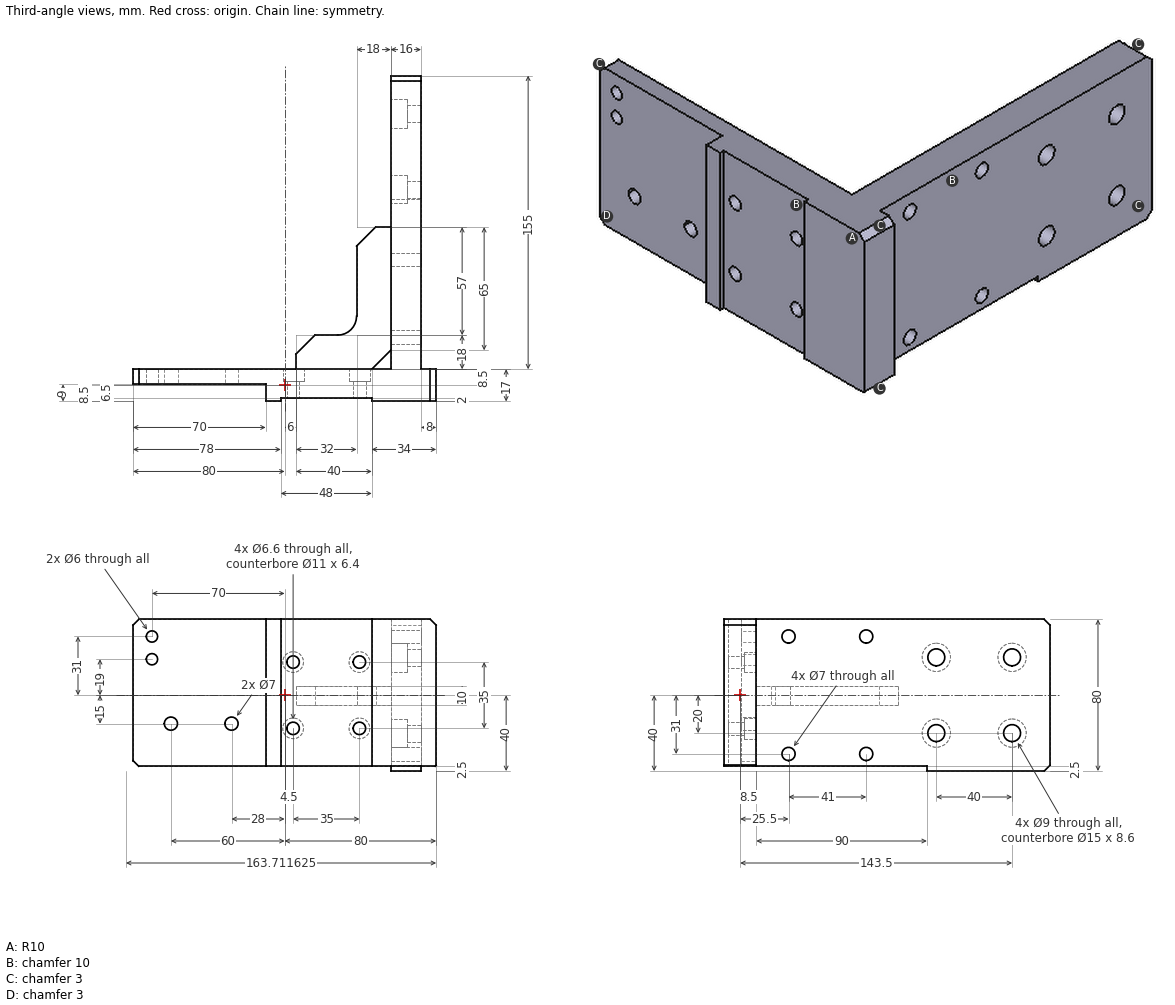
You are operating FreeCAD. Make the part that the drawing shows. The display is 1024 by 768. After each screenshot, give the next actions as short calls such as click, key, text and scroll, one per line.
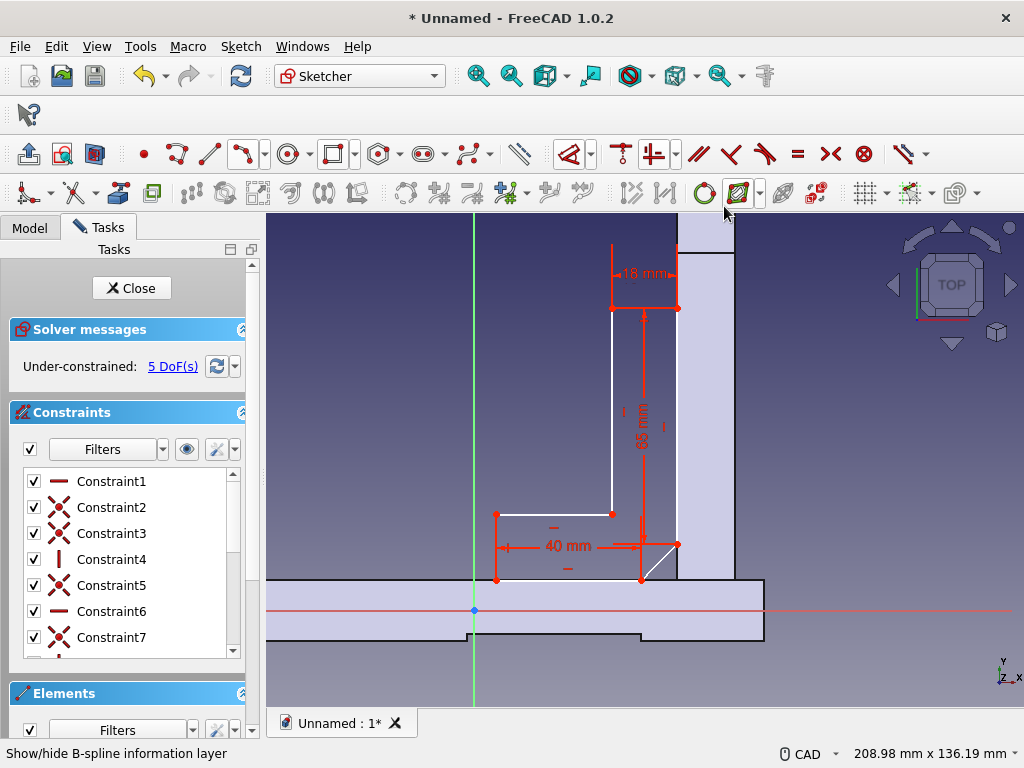
click(612, 370)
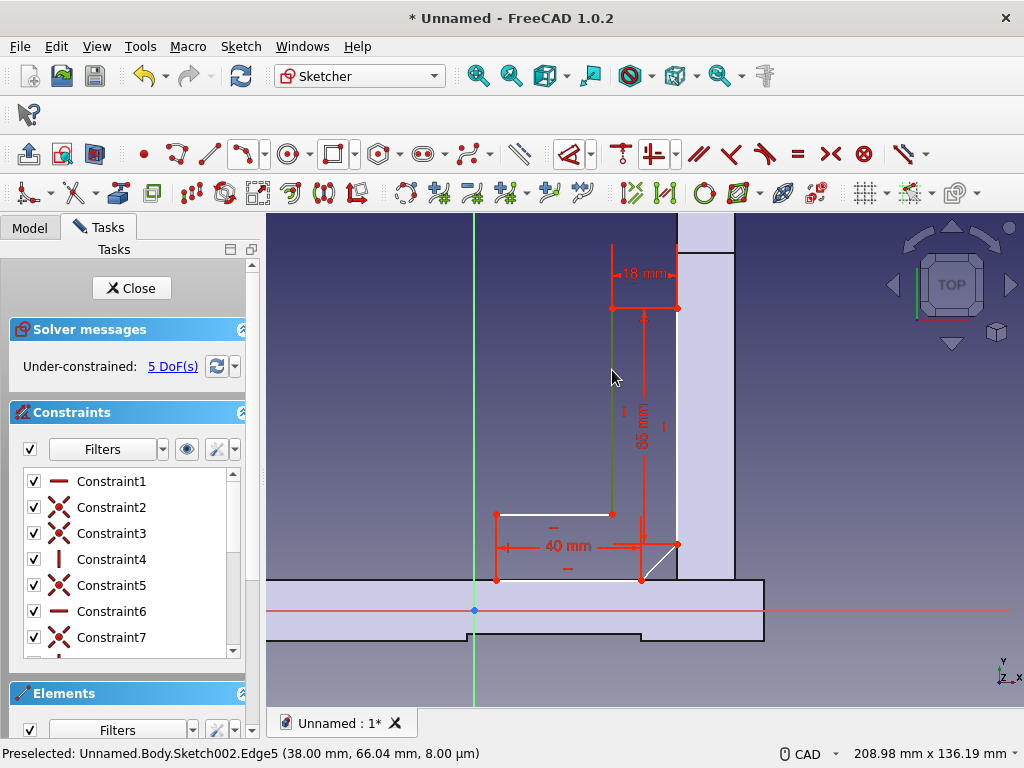
key(i)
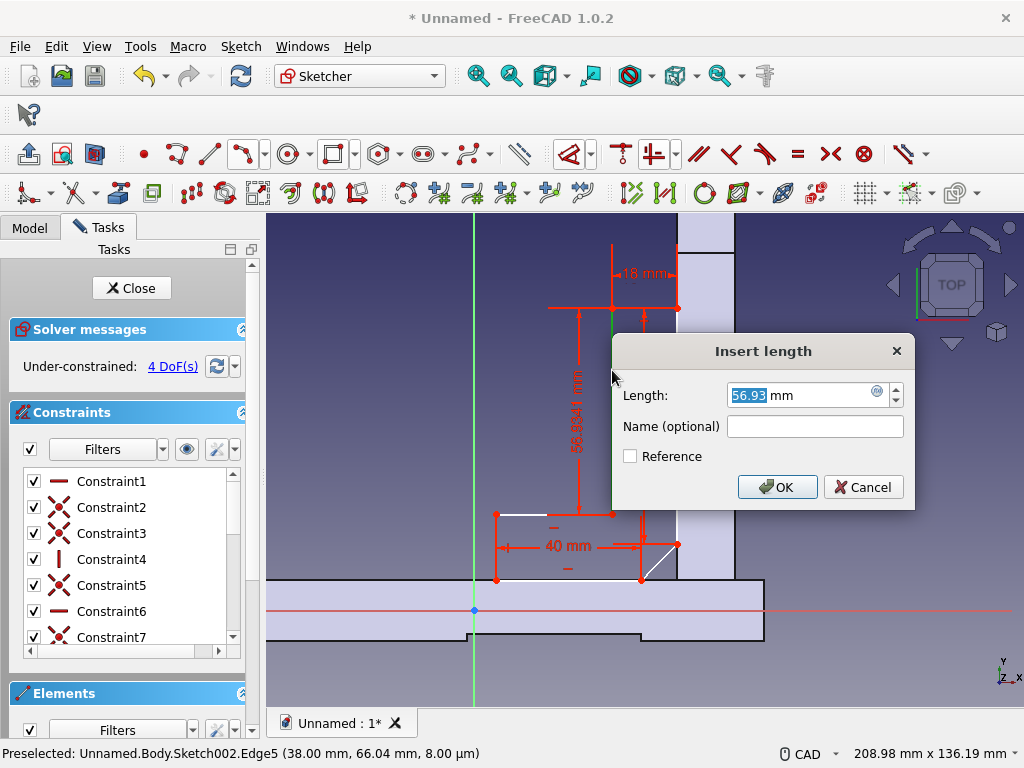
text(57)
key(Return)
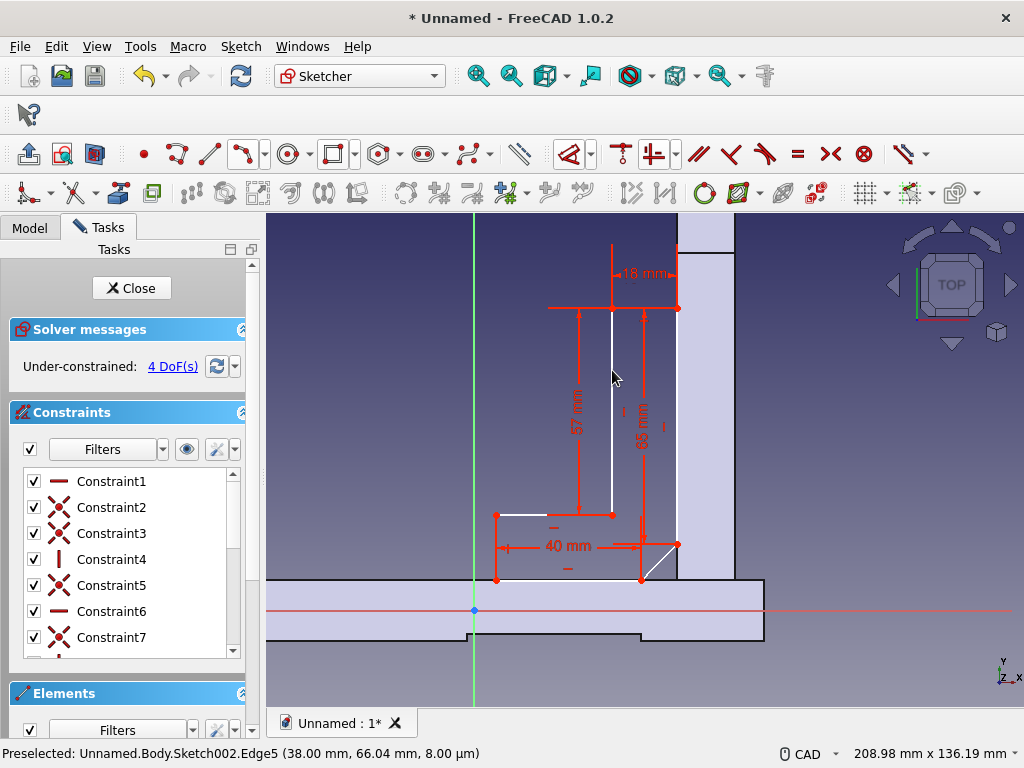
click(577, 515)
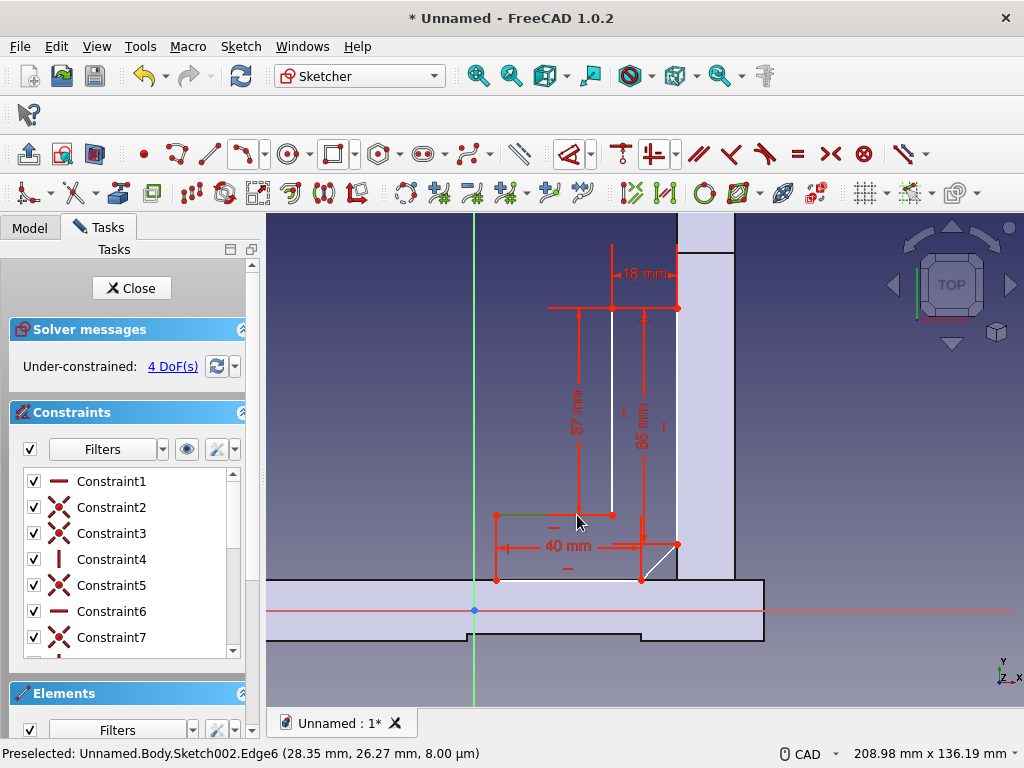
key(l)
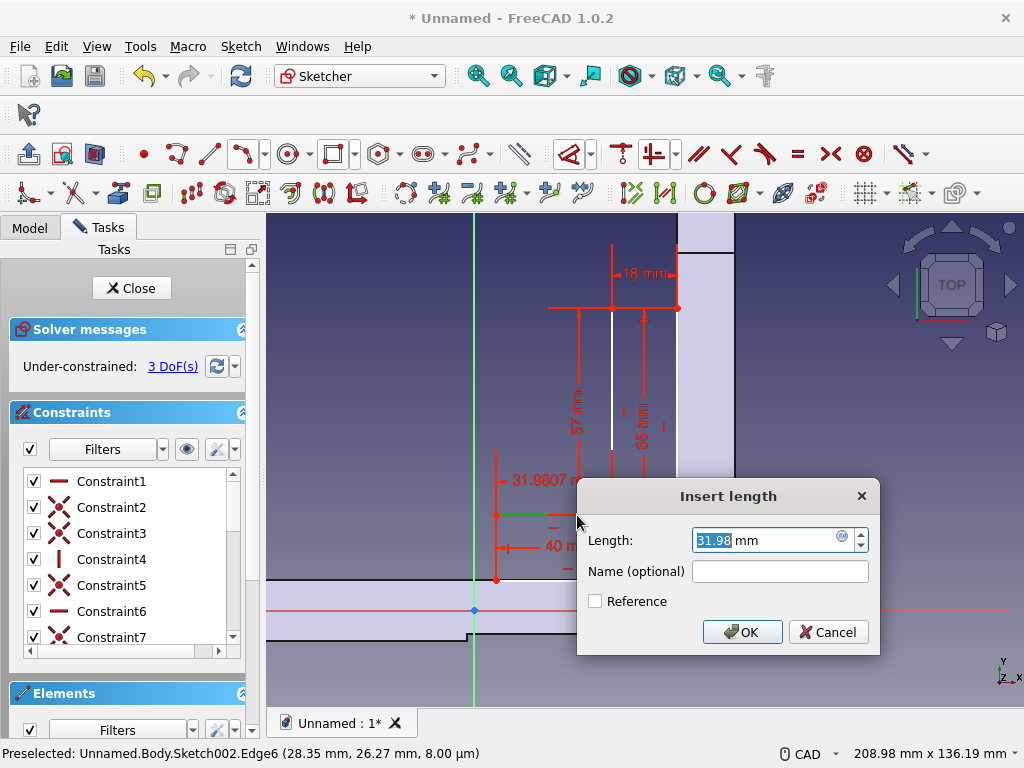
text(32)
key(Return)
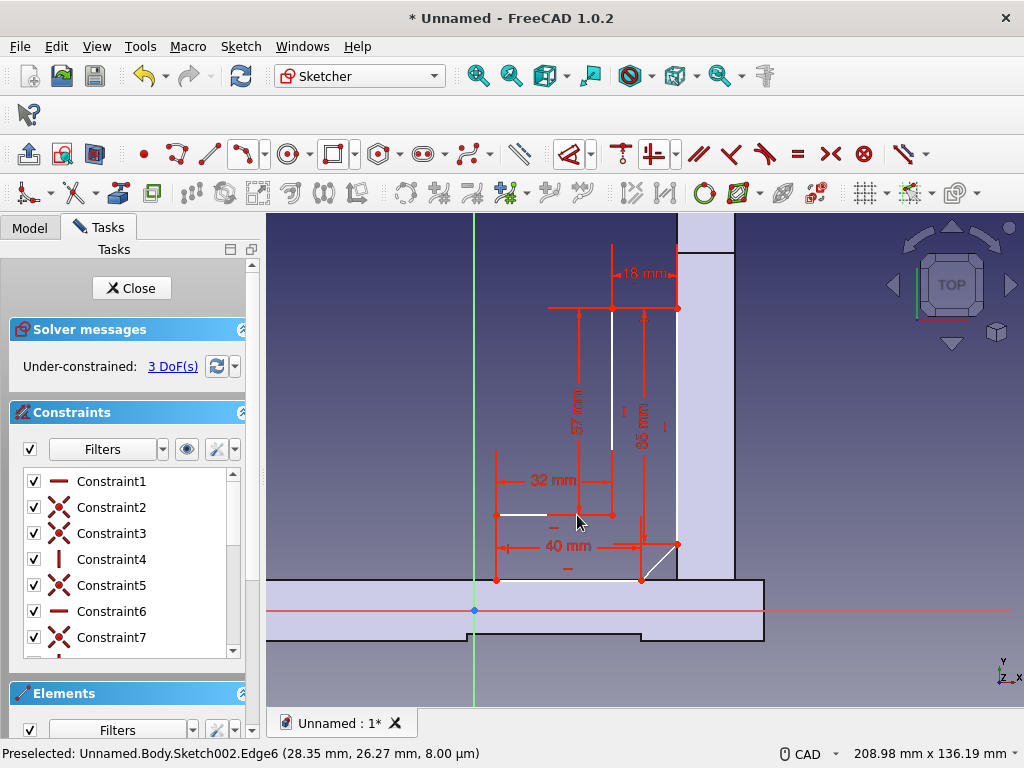
click(496, 535)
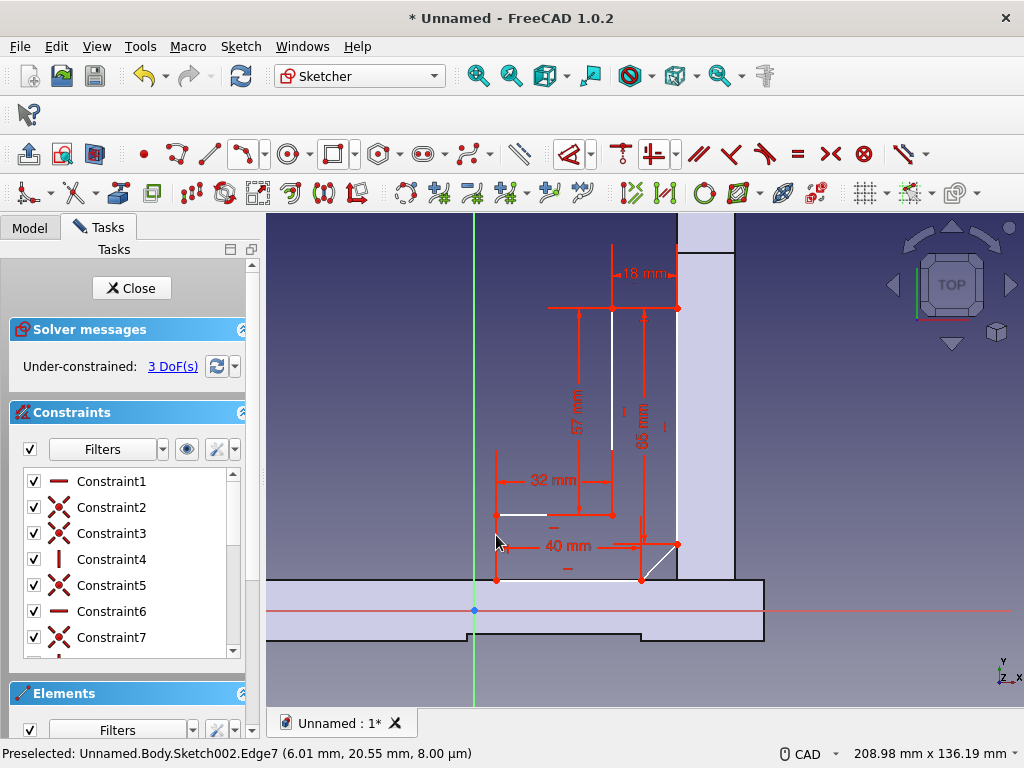
key(i)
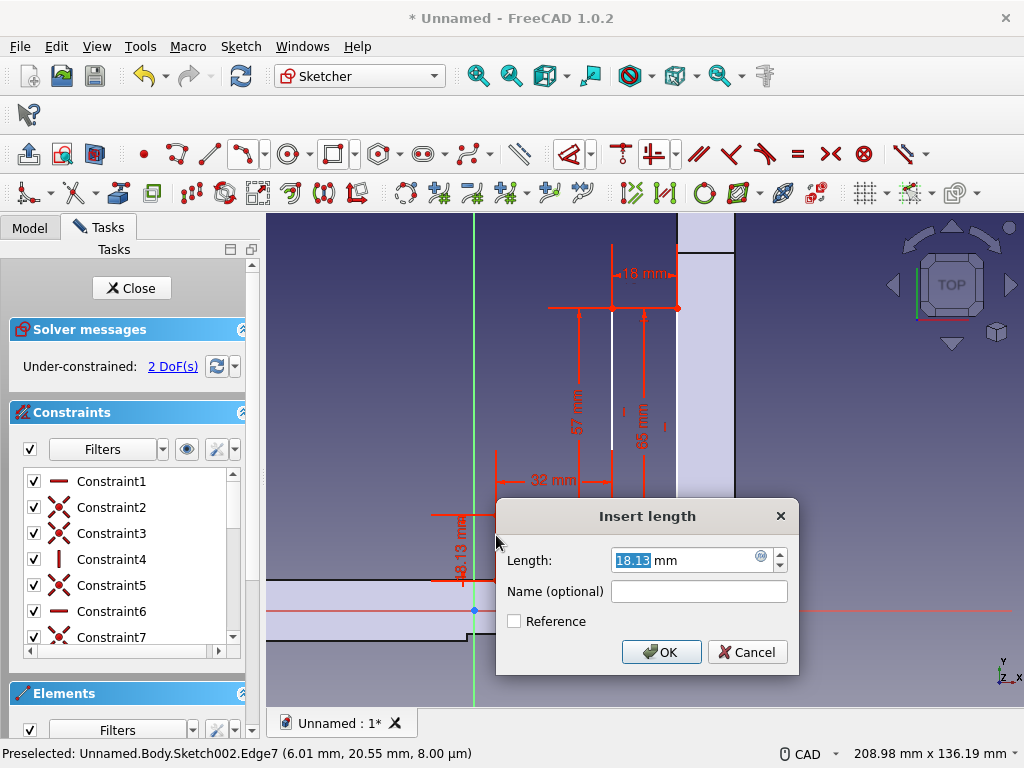
text(18)
key(Return)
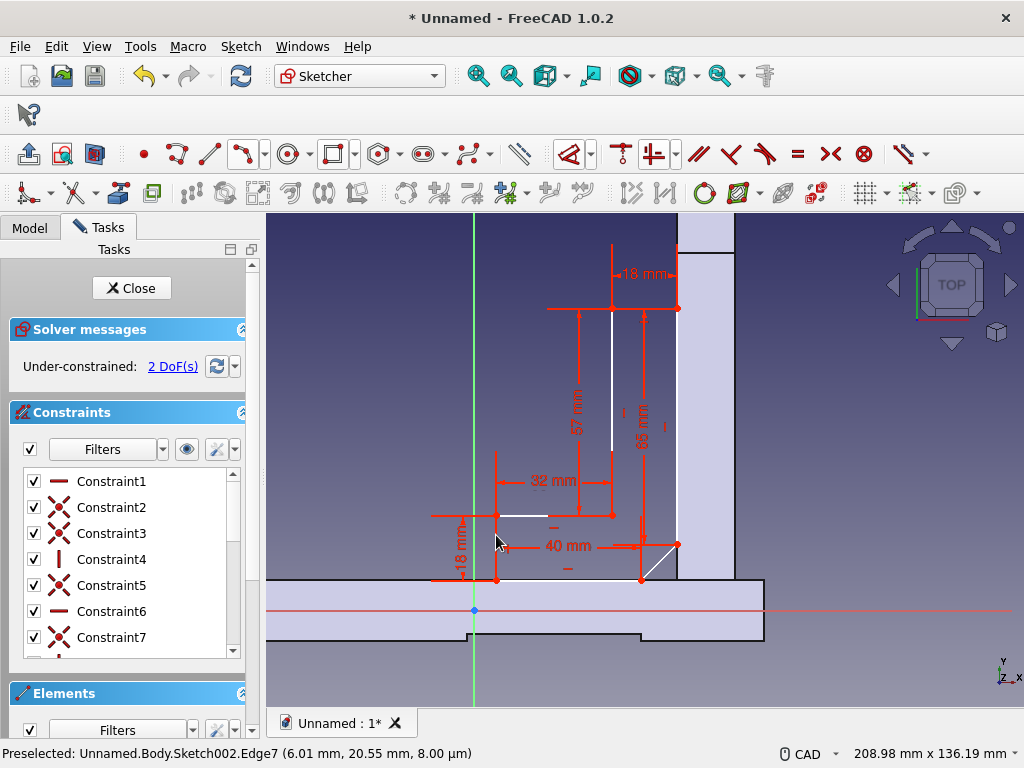
scroll(496, 581, up, 4)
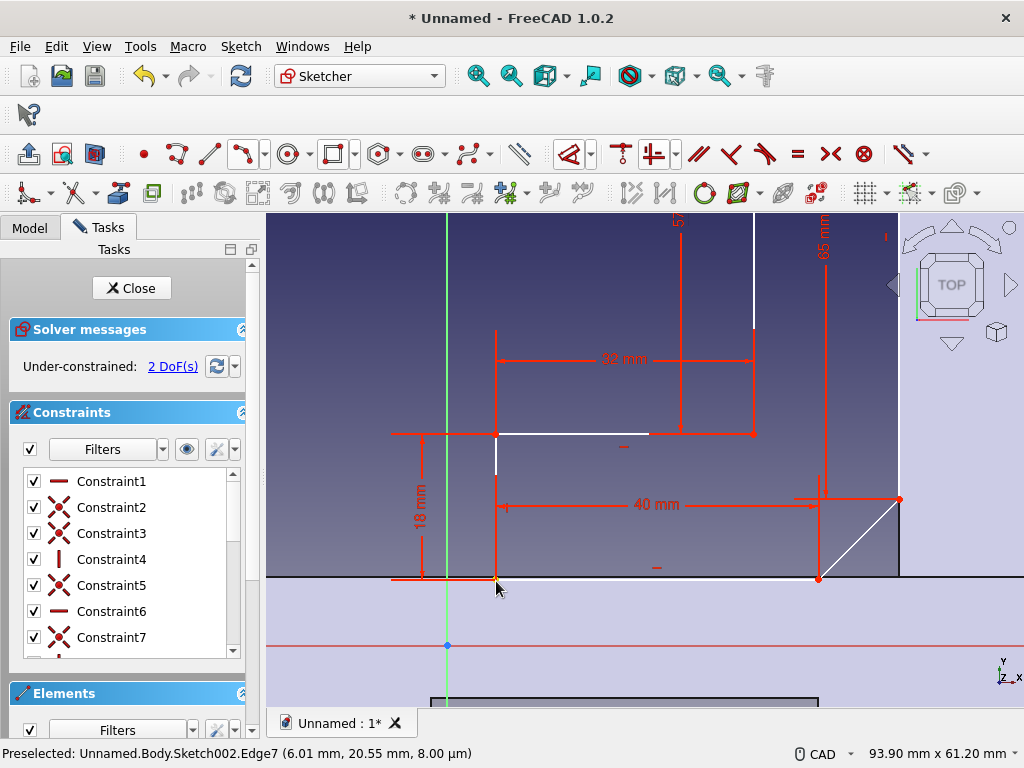
click(496, 580)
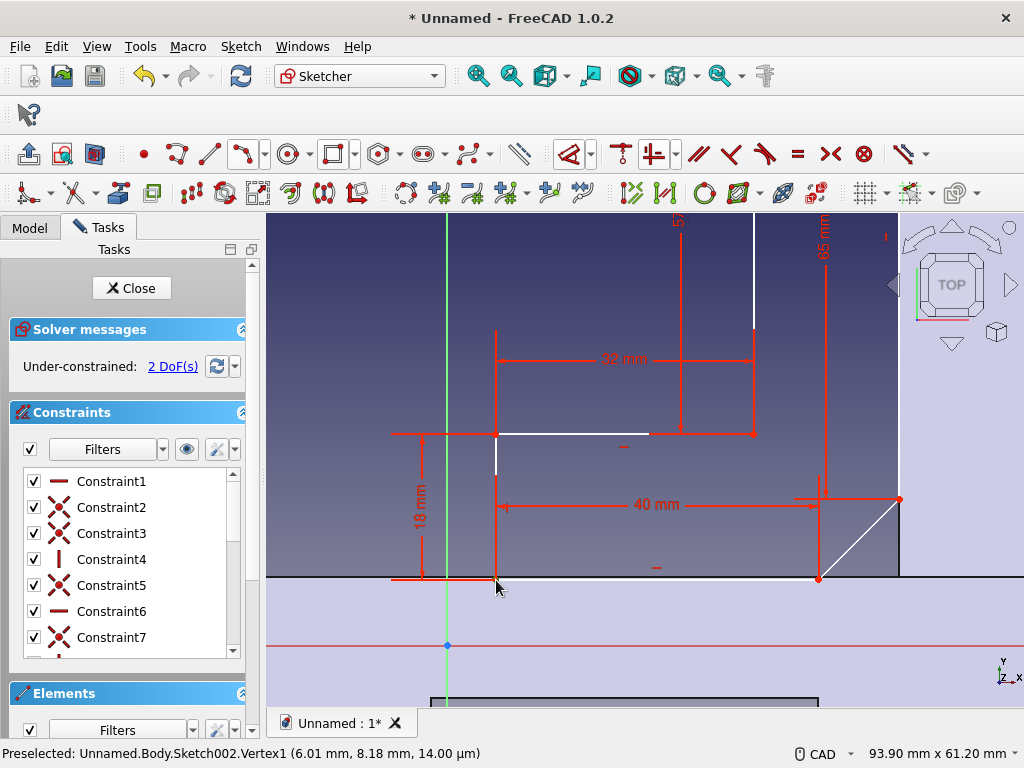
key(l)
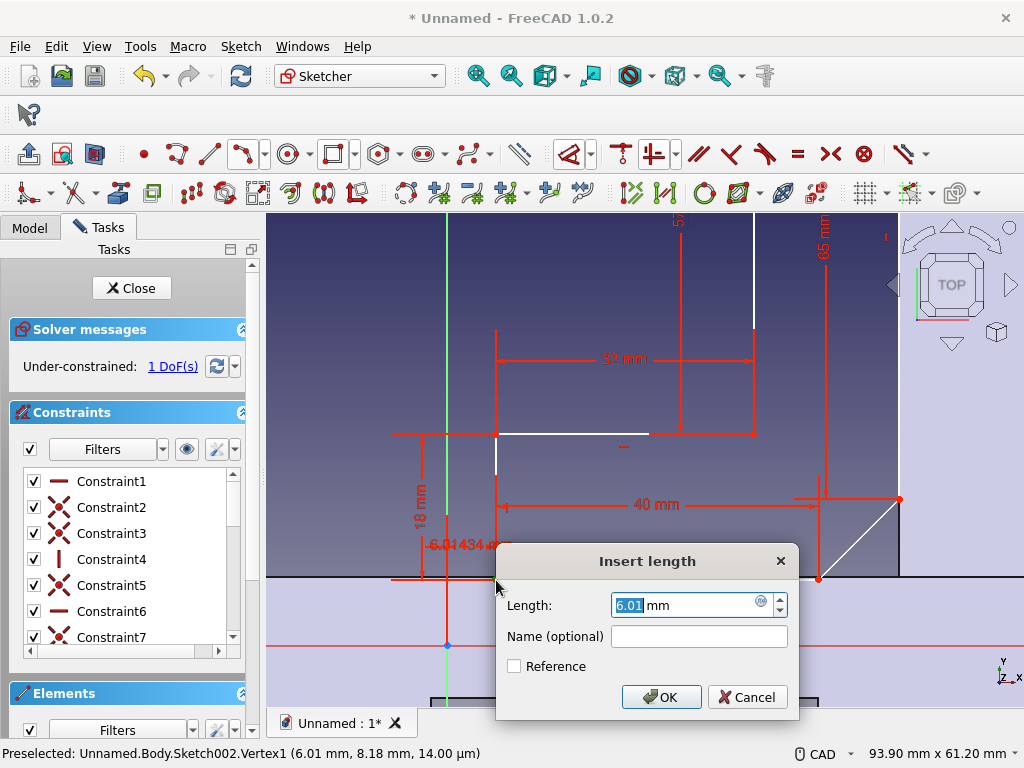
text(6)
key(Return)